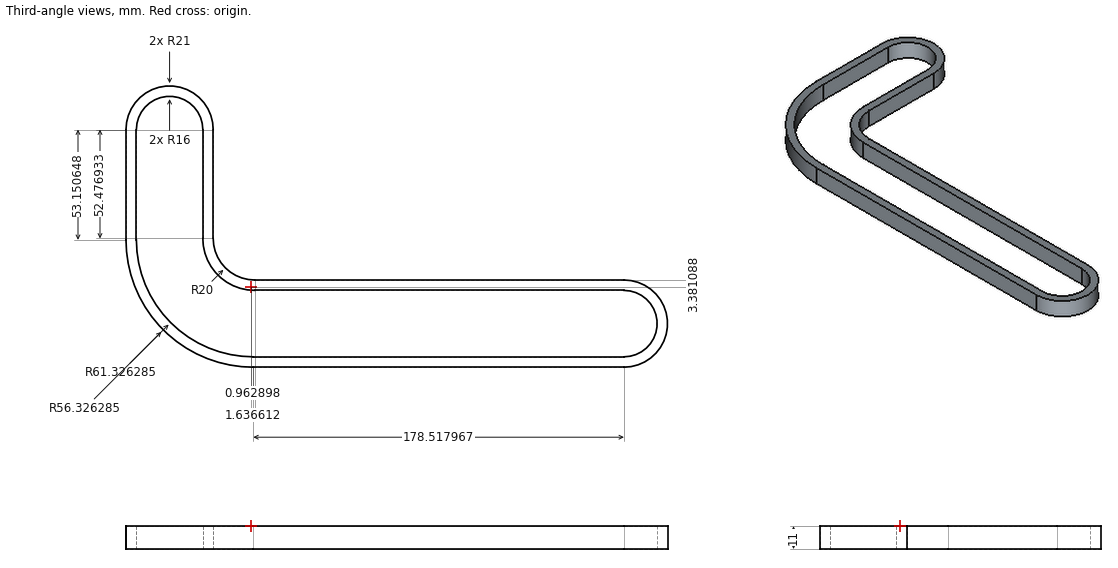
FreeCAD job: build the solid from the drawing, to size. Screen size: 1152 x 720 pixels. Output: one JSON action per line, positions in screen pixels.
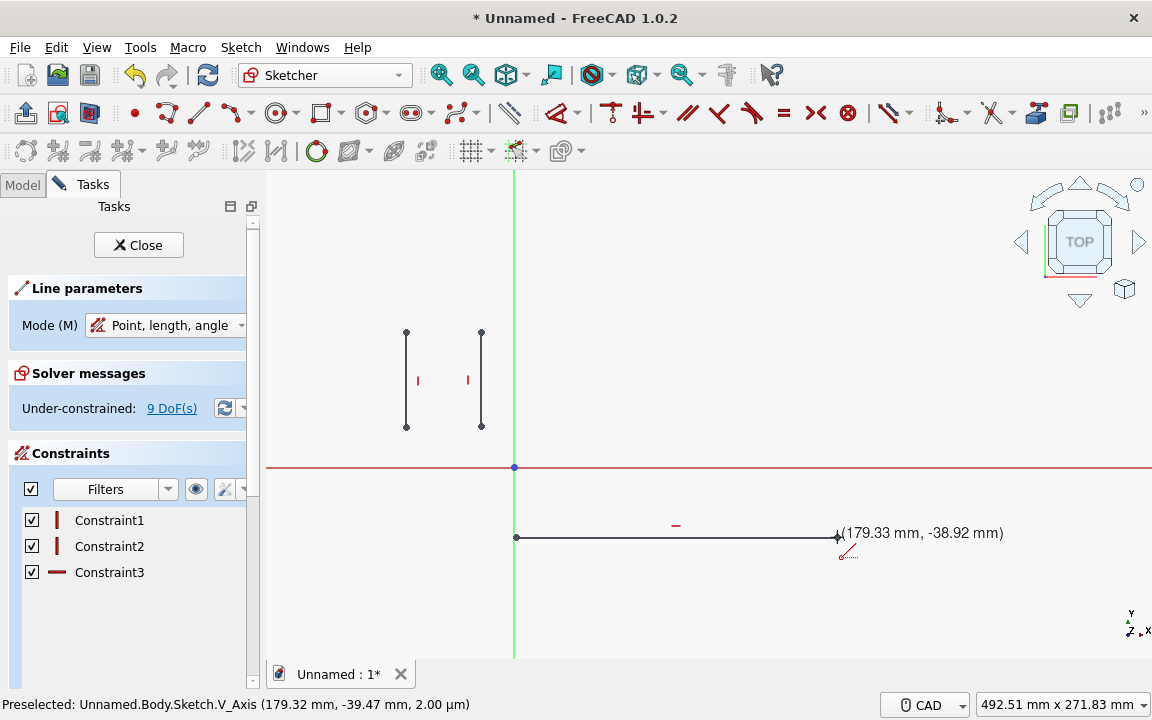
{"action": "scroll", "coordinate": [837, 462], "scroll_direction": "up", "scroll_amount": 5}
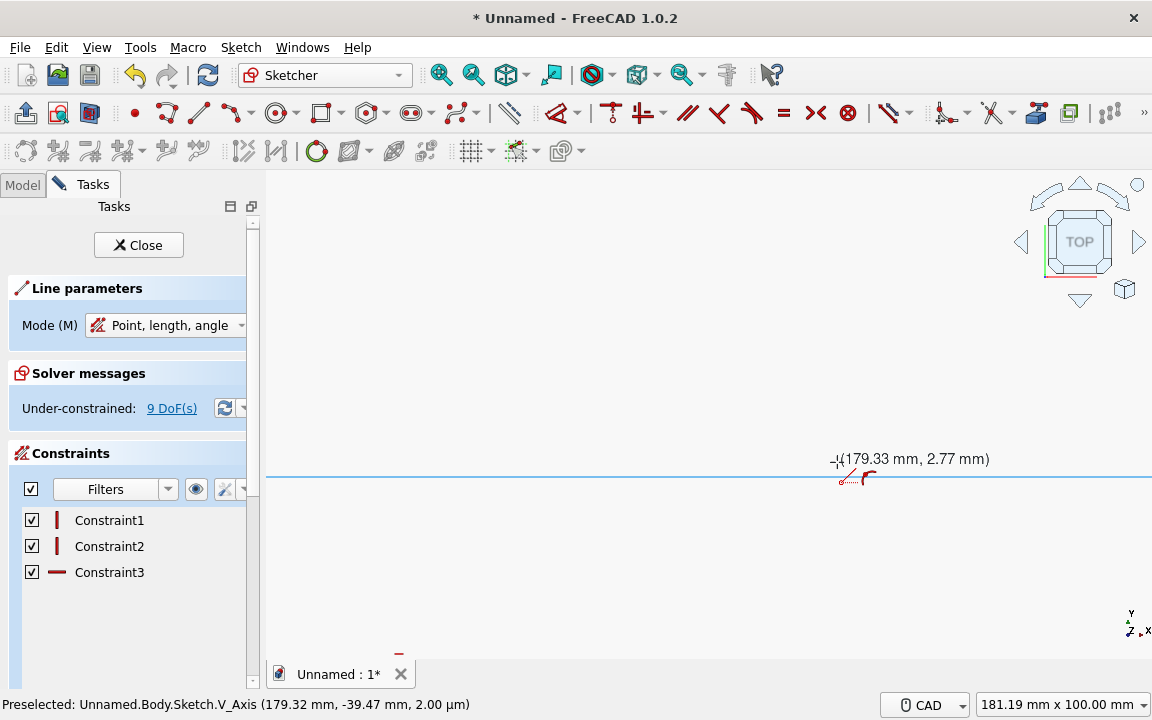
{"action": "left_click", "coordinate": [837, 461]}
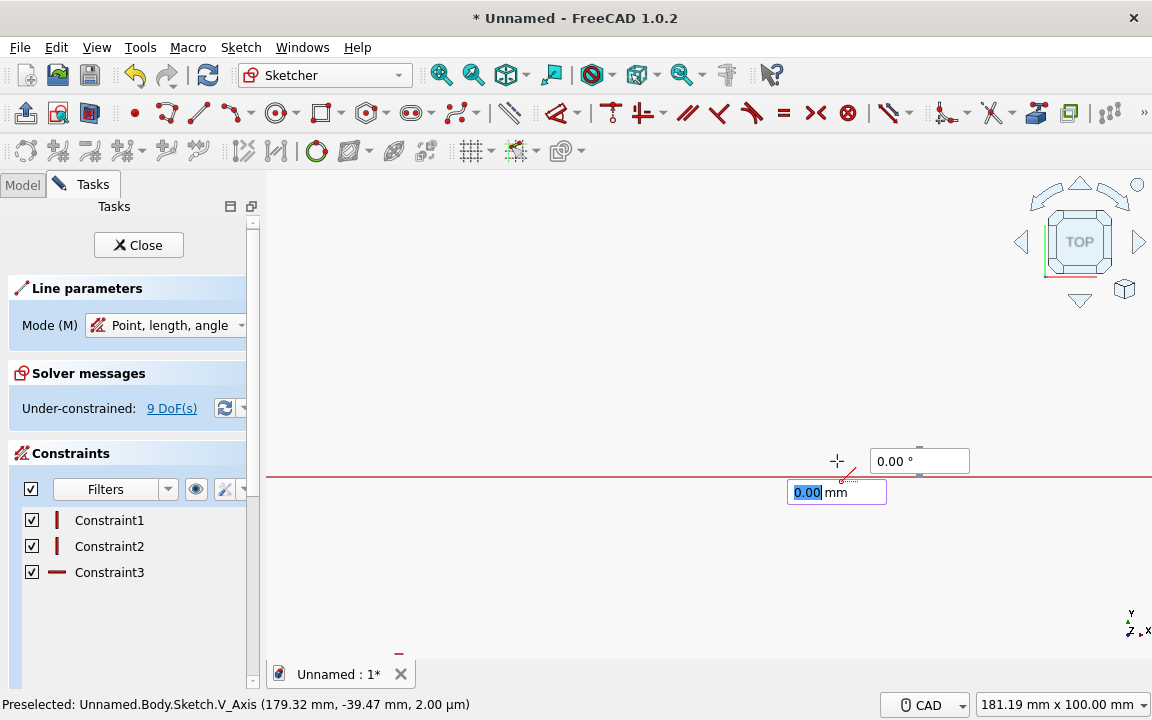
{"action": "scroll", "coordinate": [838, 461], "scroll_direction": "down", "scroll_amount": 5}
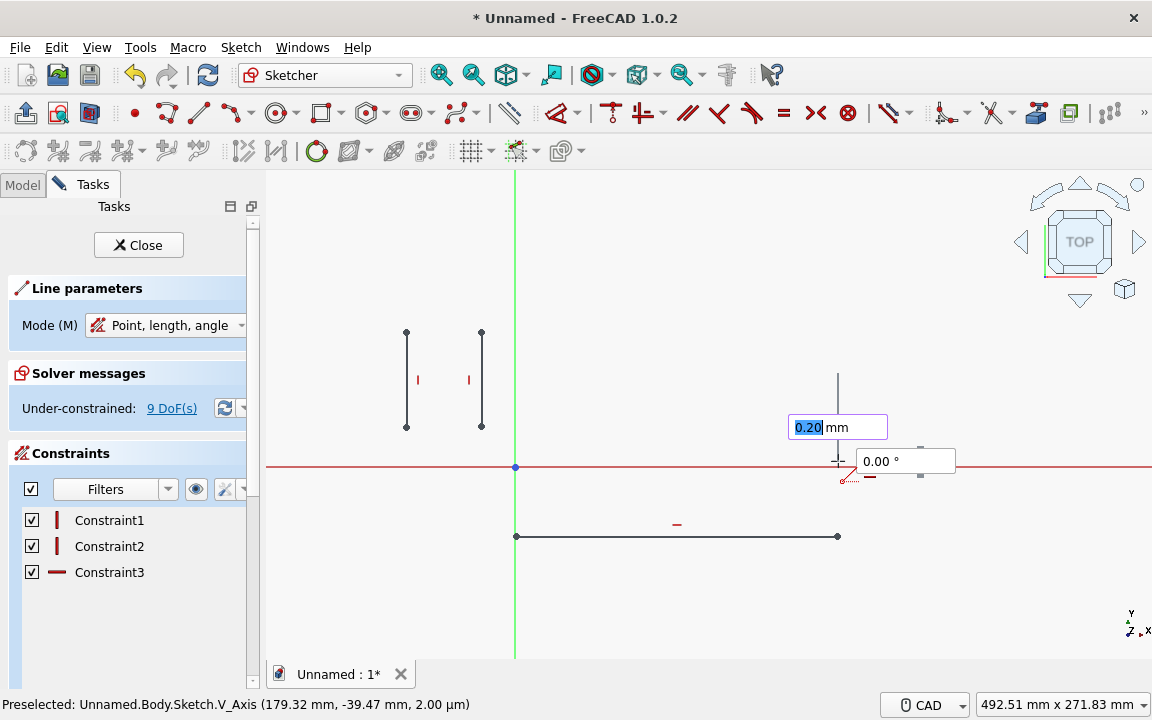
{"action": "scroll", "coordinate": [518, 461], "scroll_direction": "up", "scroll_amount": 9}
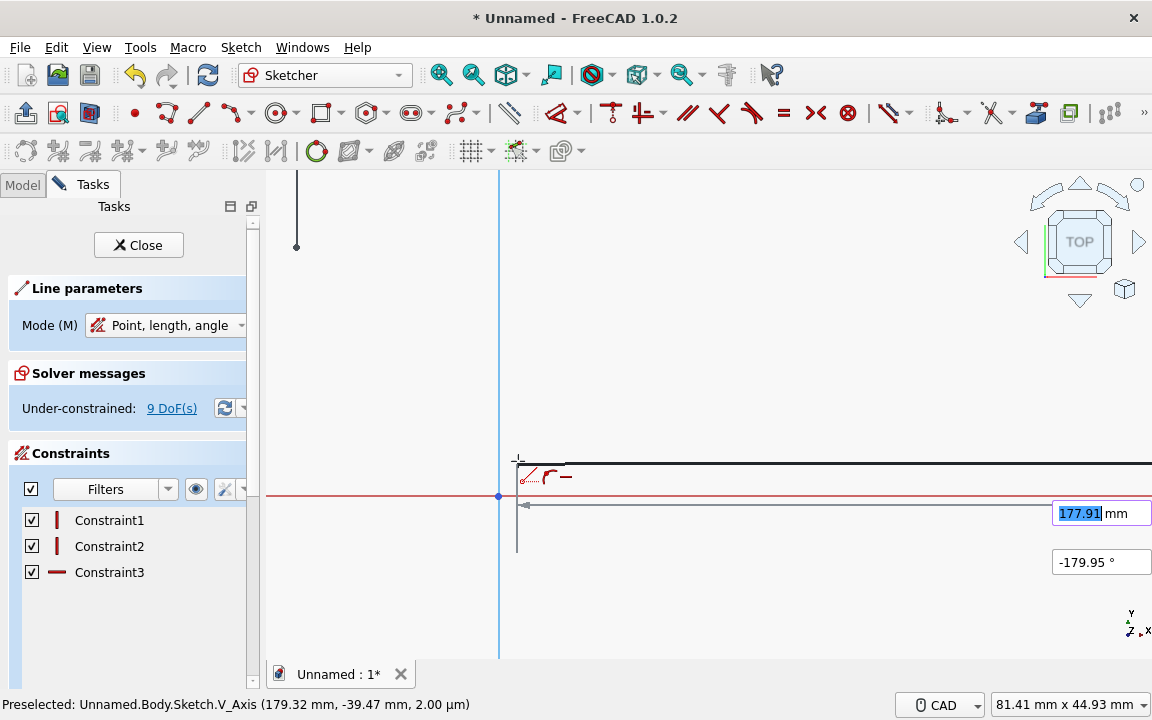
{"action": "left_click", "coordinate": [516, 460]}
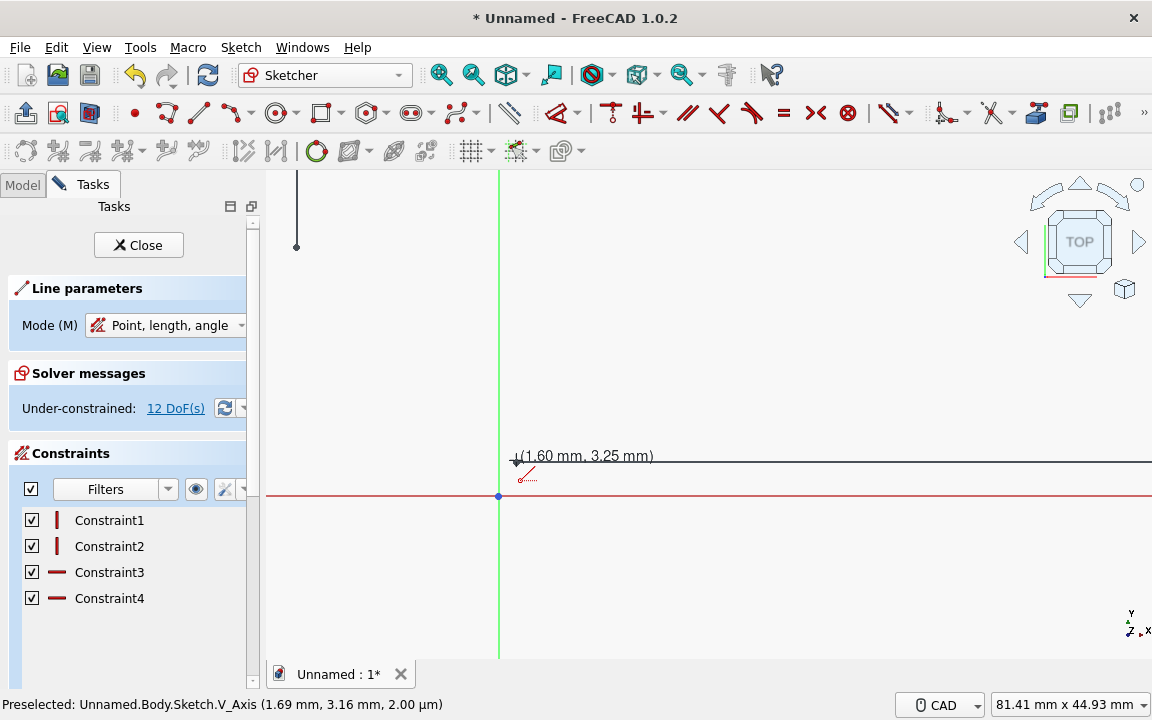
{"action": "left_click", "coordinate": [232, 114]}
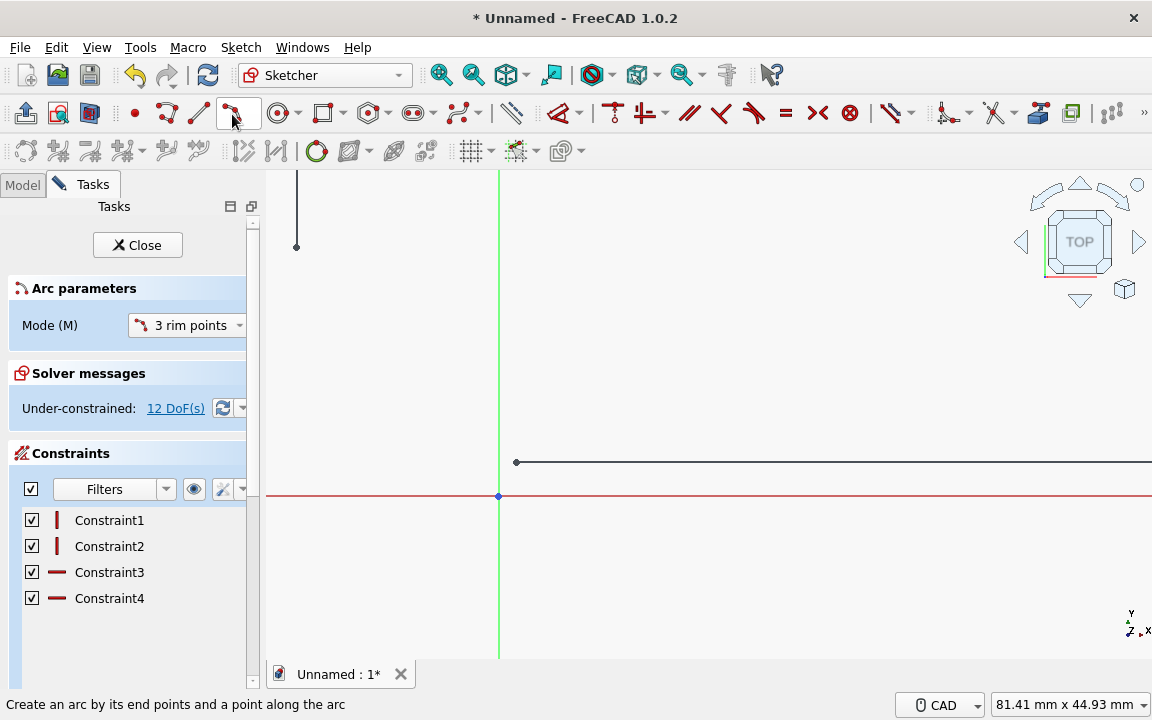
{"action": "scroll", "coordinate": [518, 461], "scroll_direction": "down", "scroll_amount": 9}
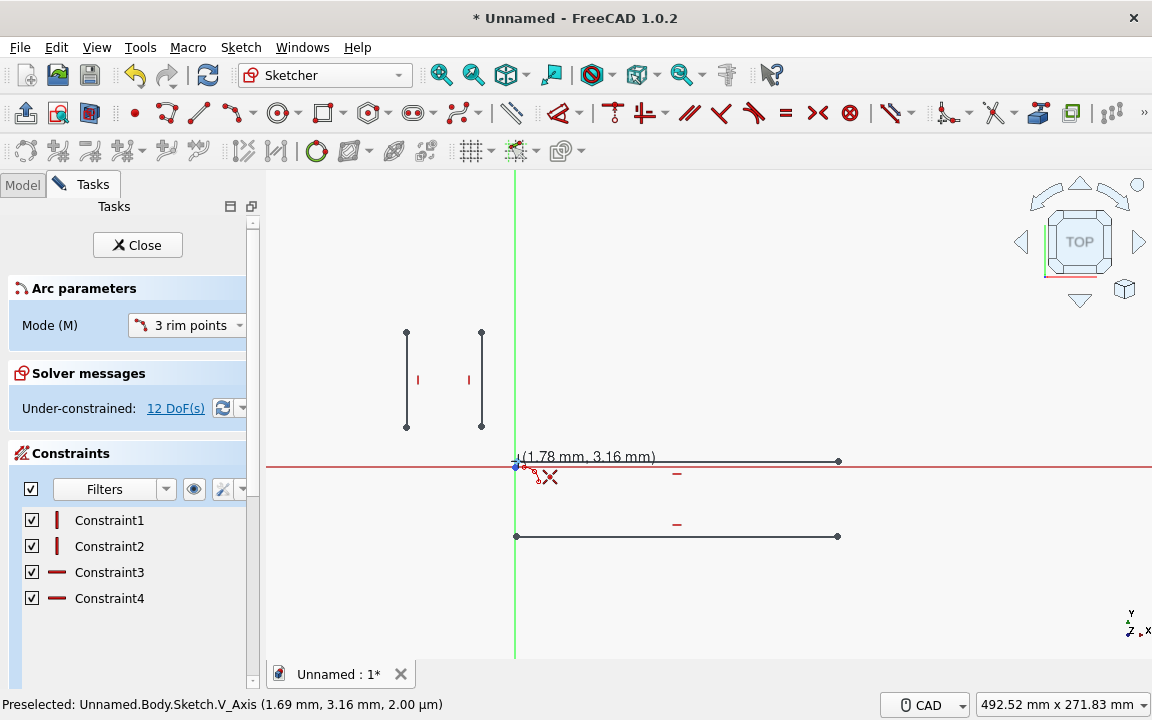
{"action": "left_click", "coordinate": [482, 332]}
{"action": "left_click", "coordinate": [407, 332]}
{"action": "left_click", "coordinate": [444, 293]}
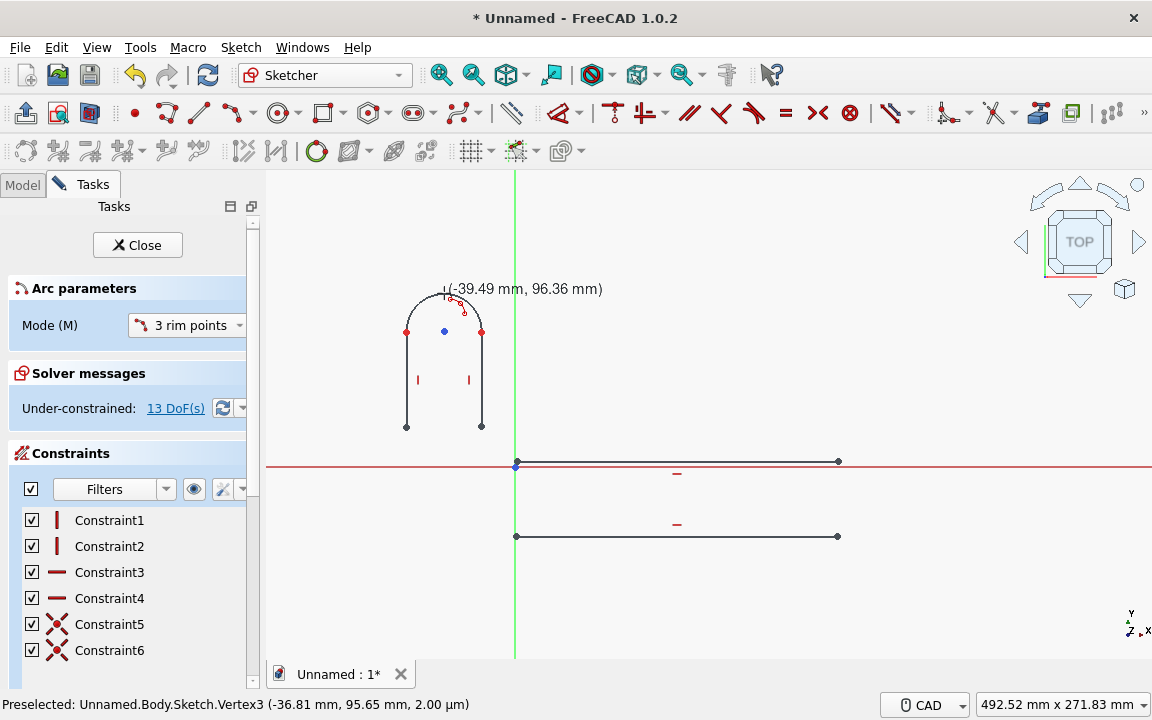
{"action": "left_click", "coordinate": [407, 427]}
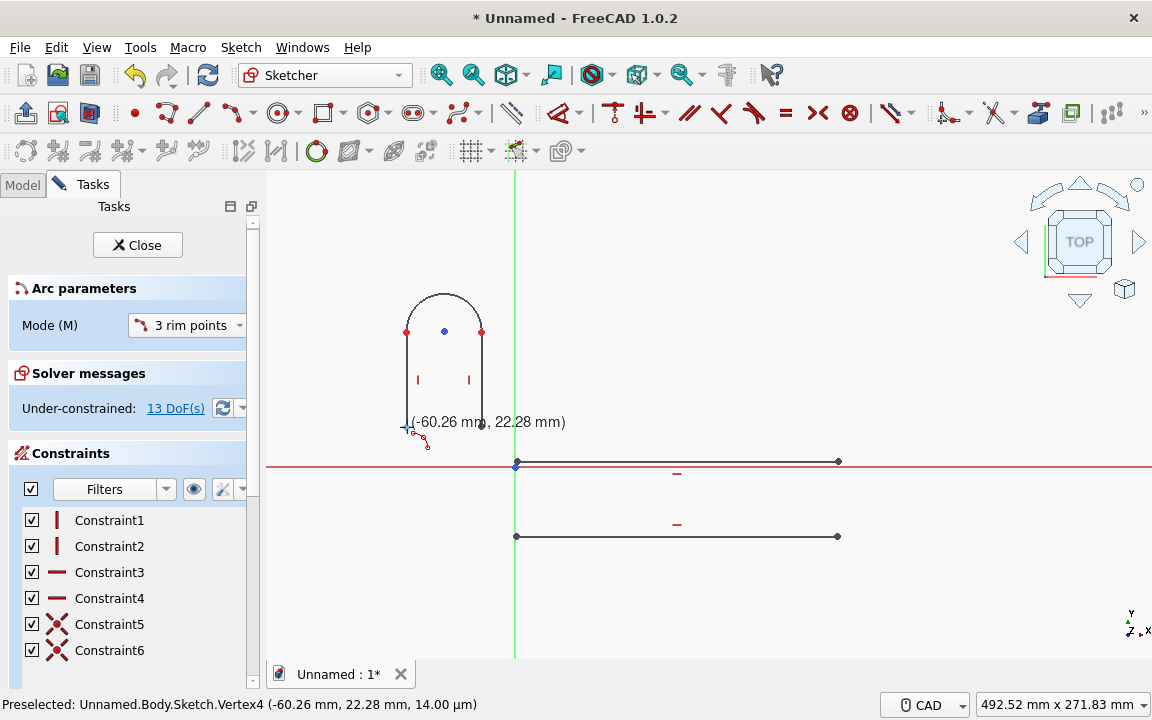
{"action": "scroll", "coordinate": [517, 537], "scroll_direction": "up", "scroll_amount": 12}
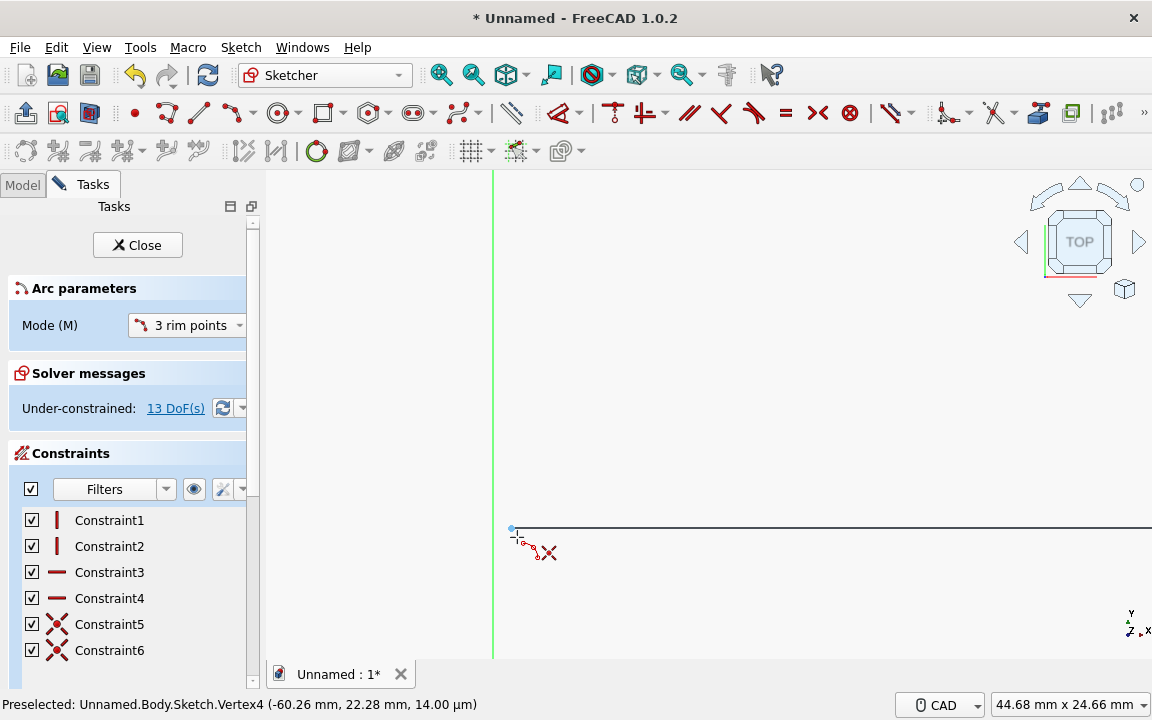
{"action": "left_click", "coordinate": [512, 528]}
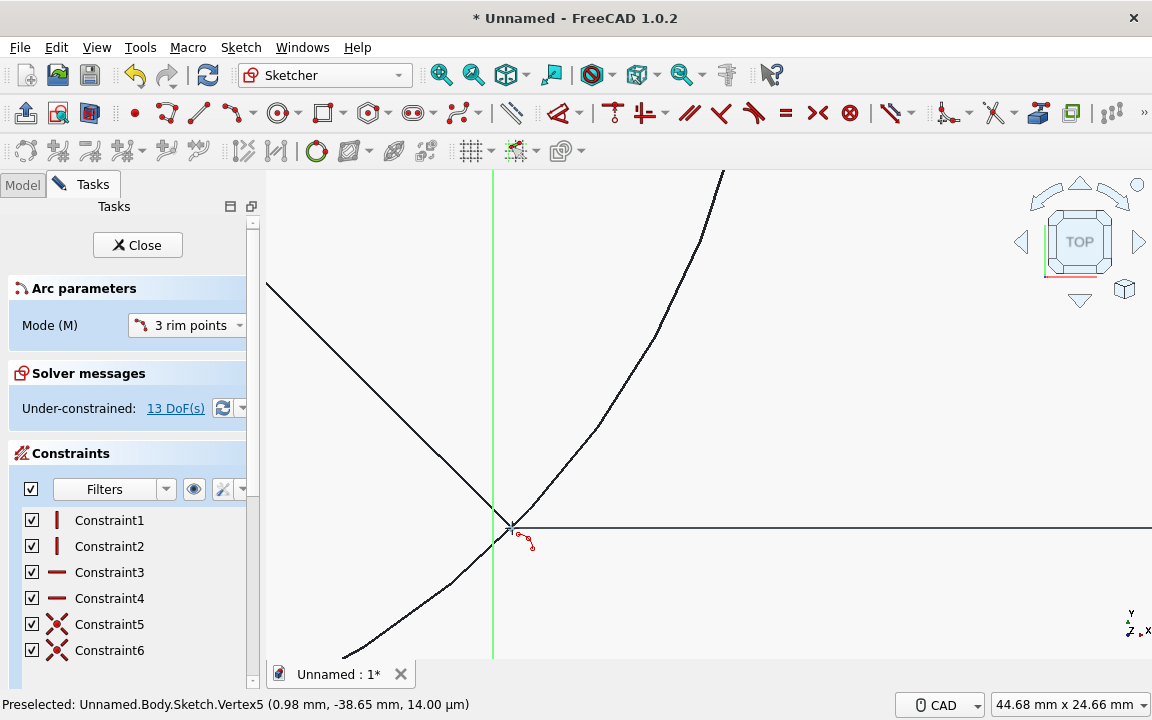
{"action": "scroll", "coordinate": [517, 537], "scroll_direction": "down", "scroll_amount": 12}